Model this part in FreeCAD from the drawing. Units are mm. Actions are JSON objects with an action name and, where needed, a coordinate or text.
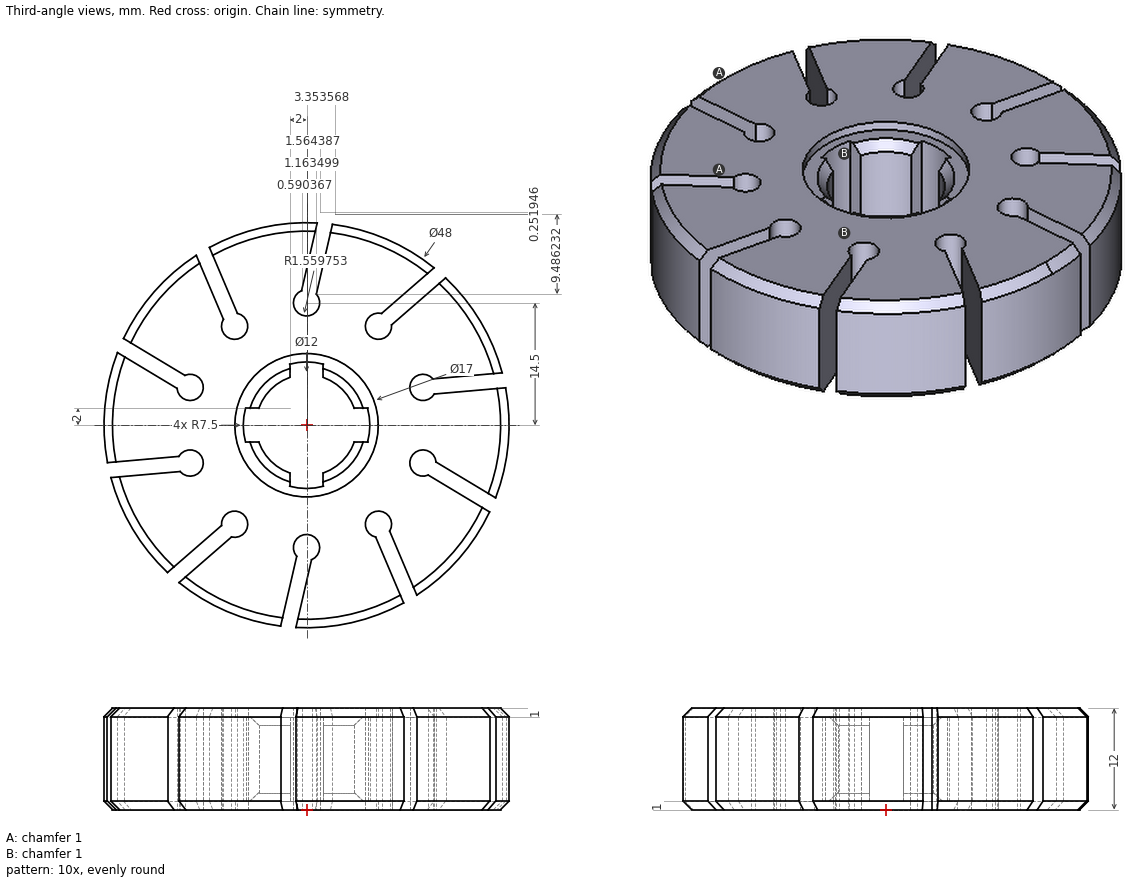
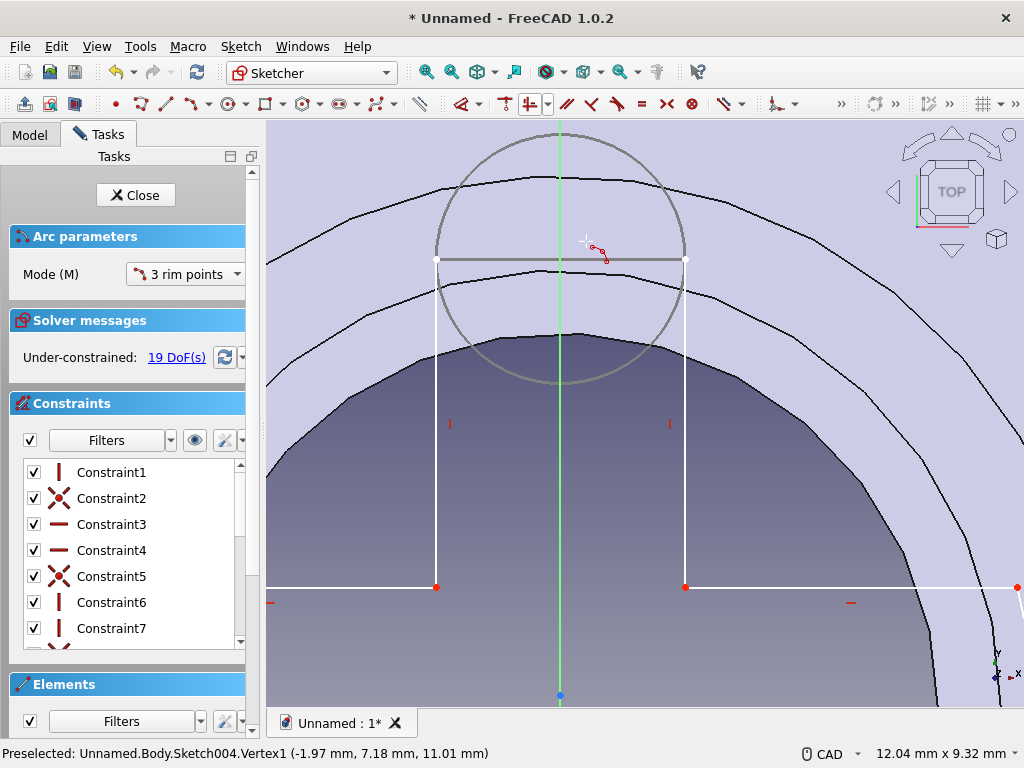
{"action": "left_click", "coordinate": [586, 240]}
{"action": "key", "text": "Escape"}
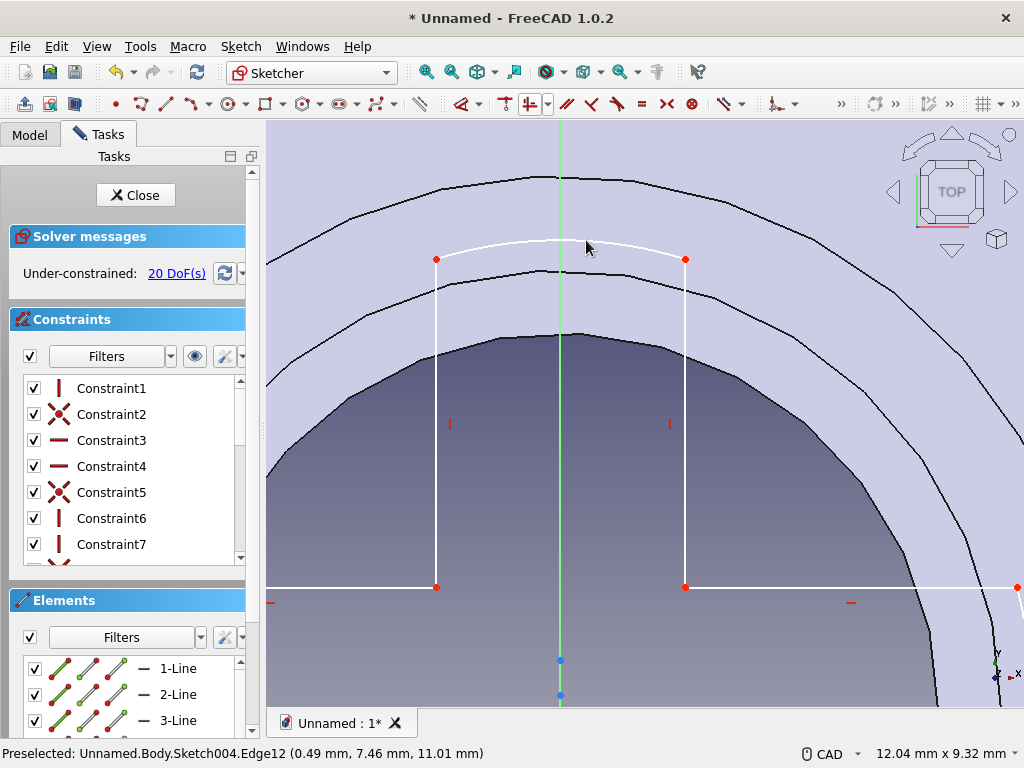
{"action": "scroll", "coordinate": [586, 240], "scroll_direction": "down", "scroll_amount": 5}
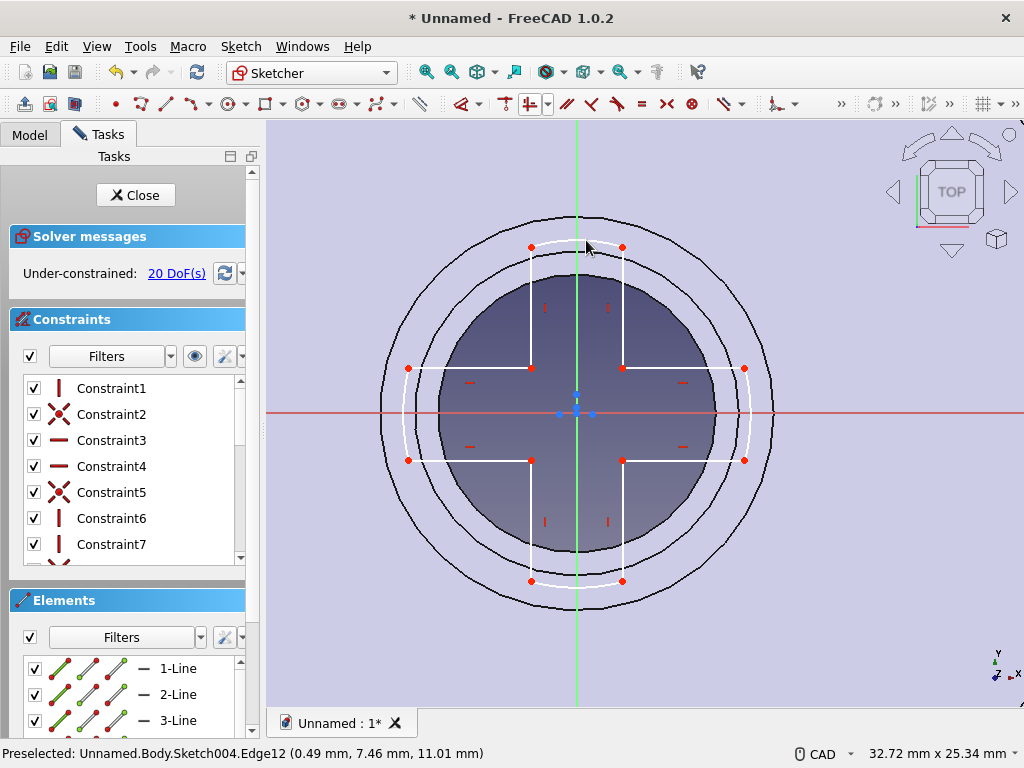
{"action": "left_click", "coordinate": [404, 396]}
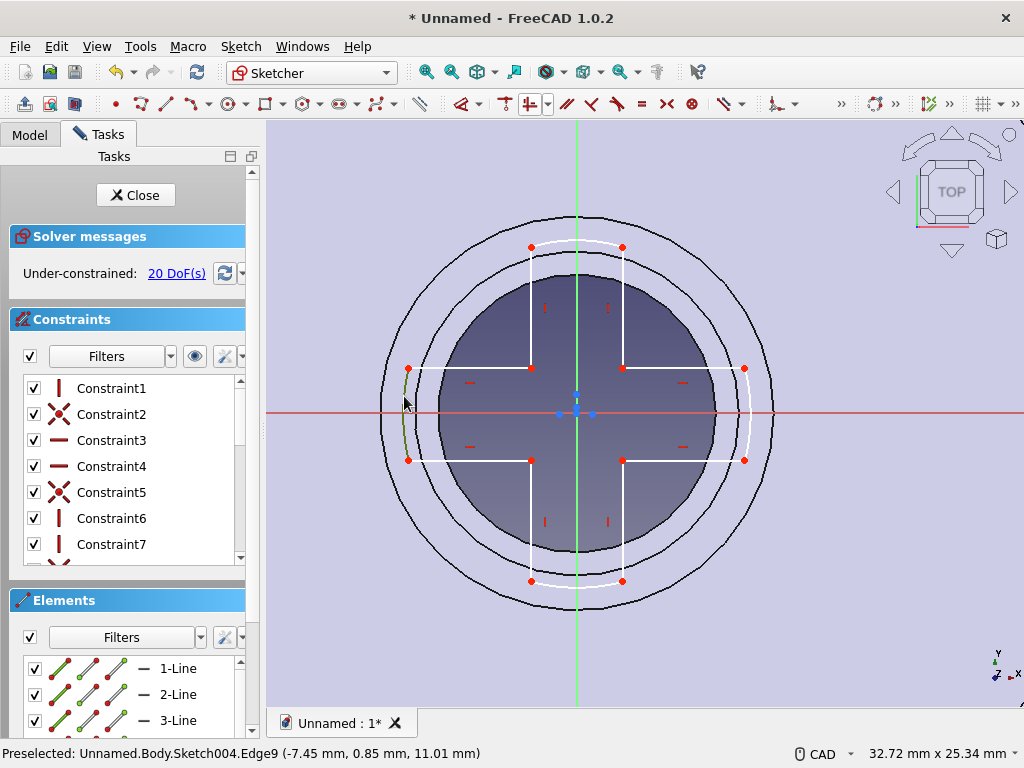
{"action": "left_click", "coordinate": [558, 587]}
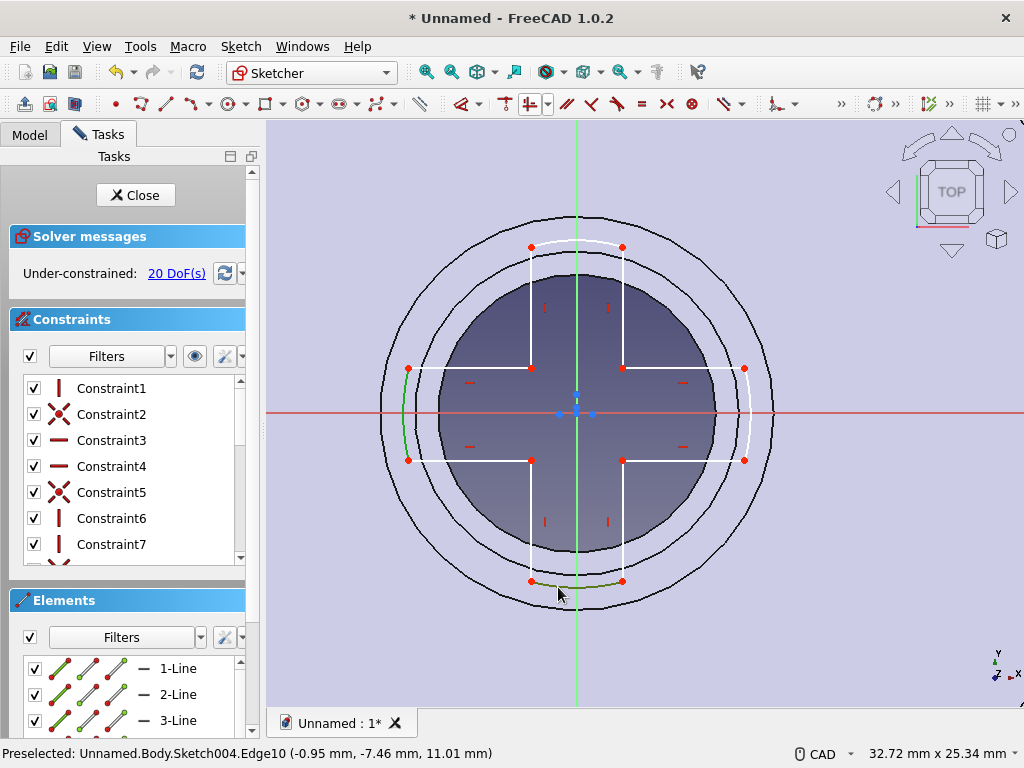
{"action": "left_click", "coordinate": [505, 104]}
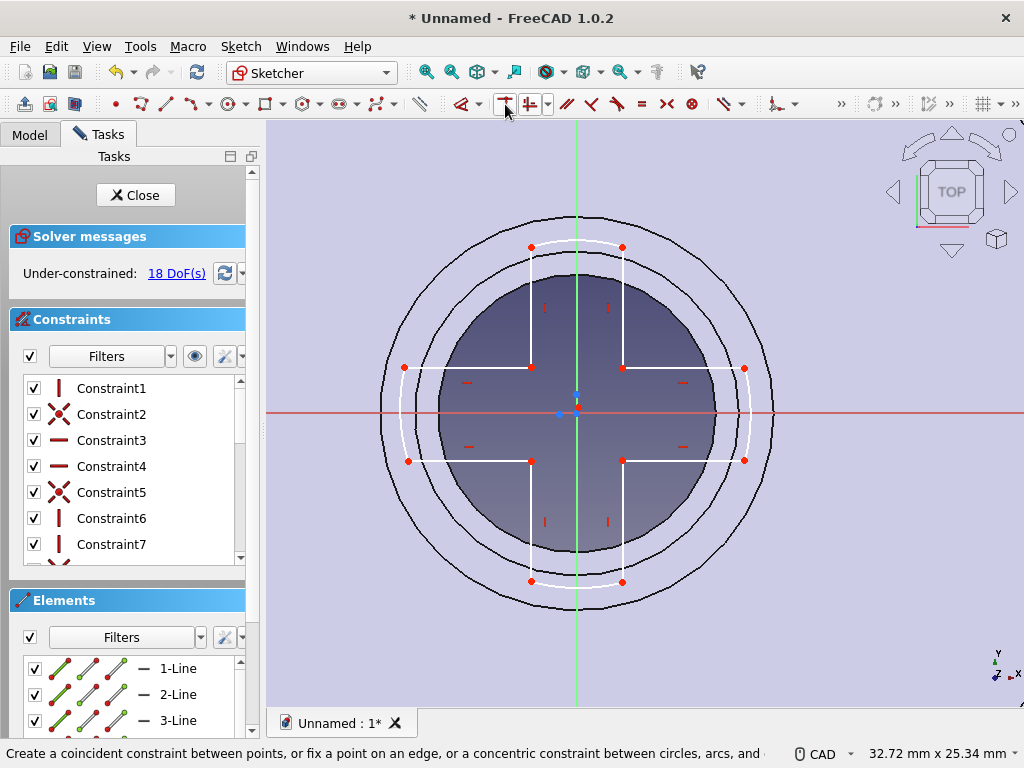
{"action": "left_click", "coordinate": [401, 396]}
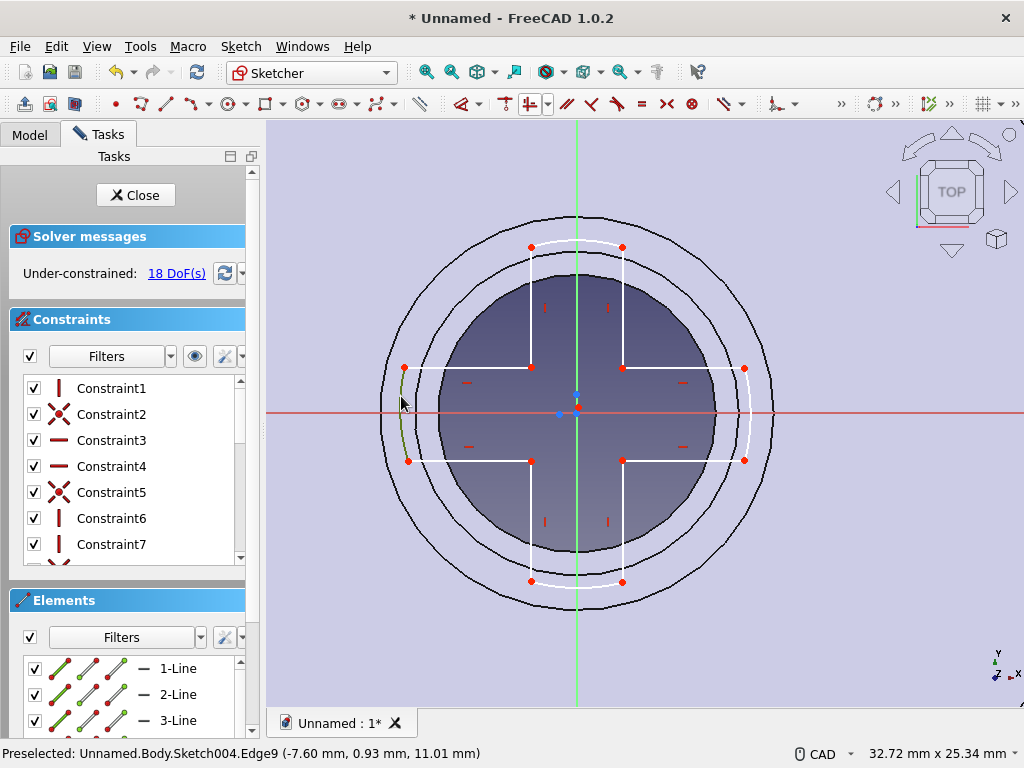
{"action": "left_click", "coordinate": [750, 433]}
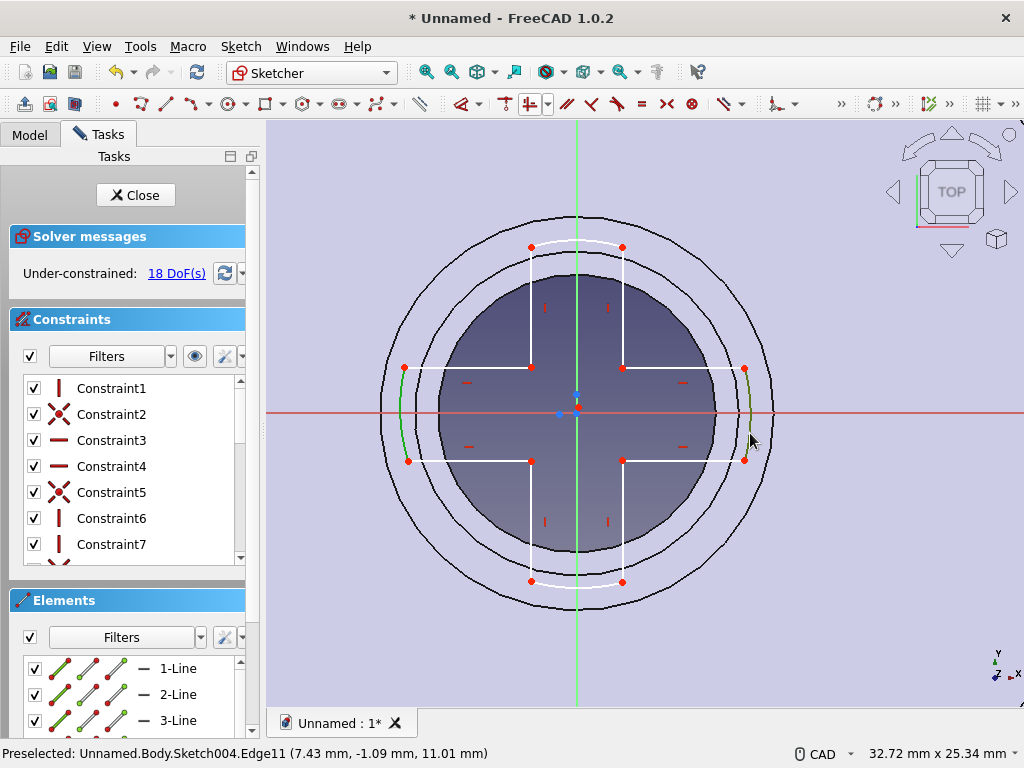
{"action": "left_click", "coordinate": [505, 104]}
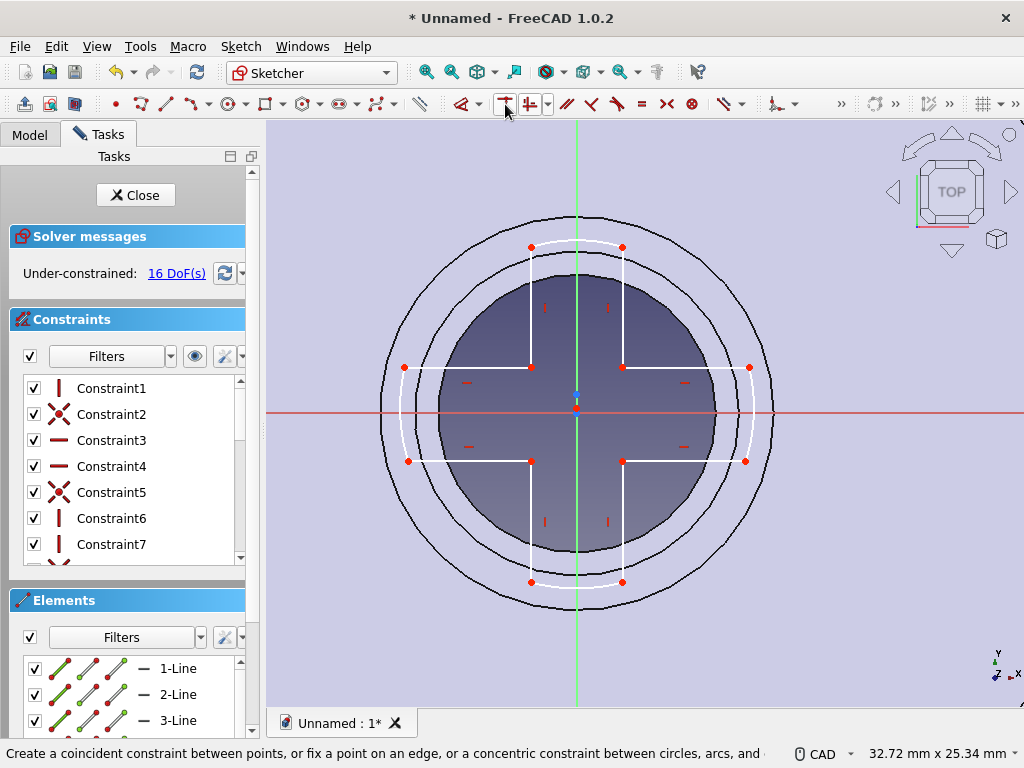
{"action": "left_click", "coordinate": [401, 396]}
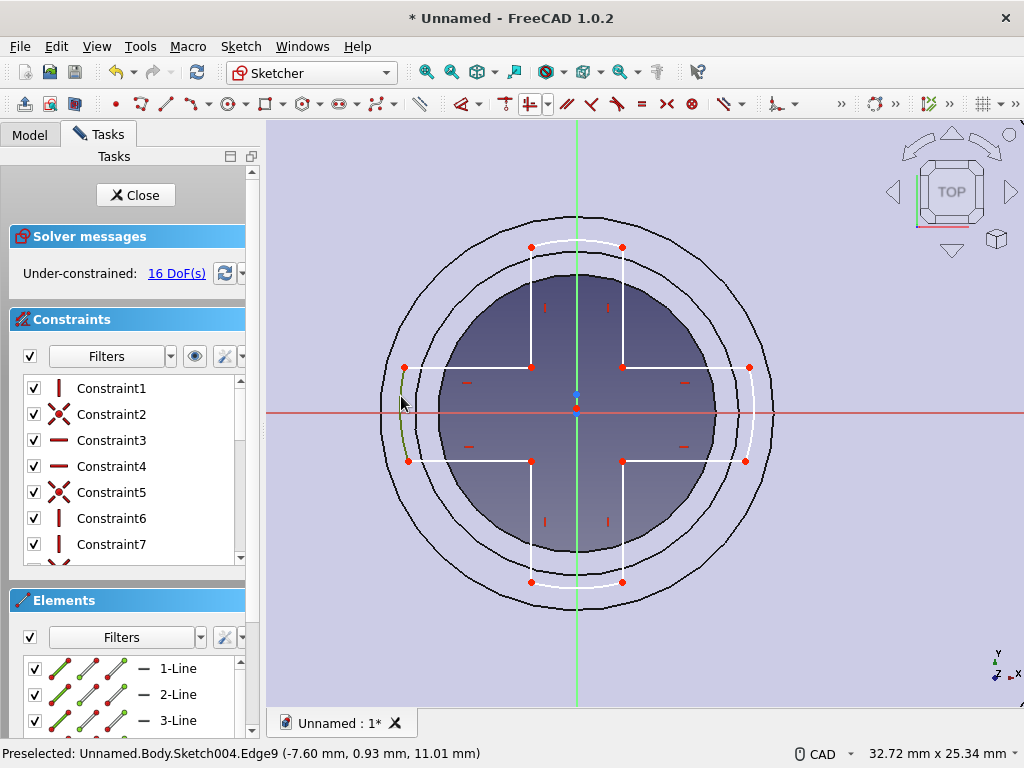
{"action": "left_click", "coordinate": [595, 241]}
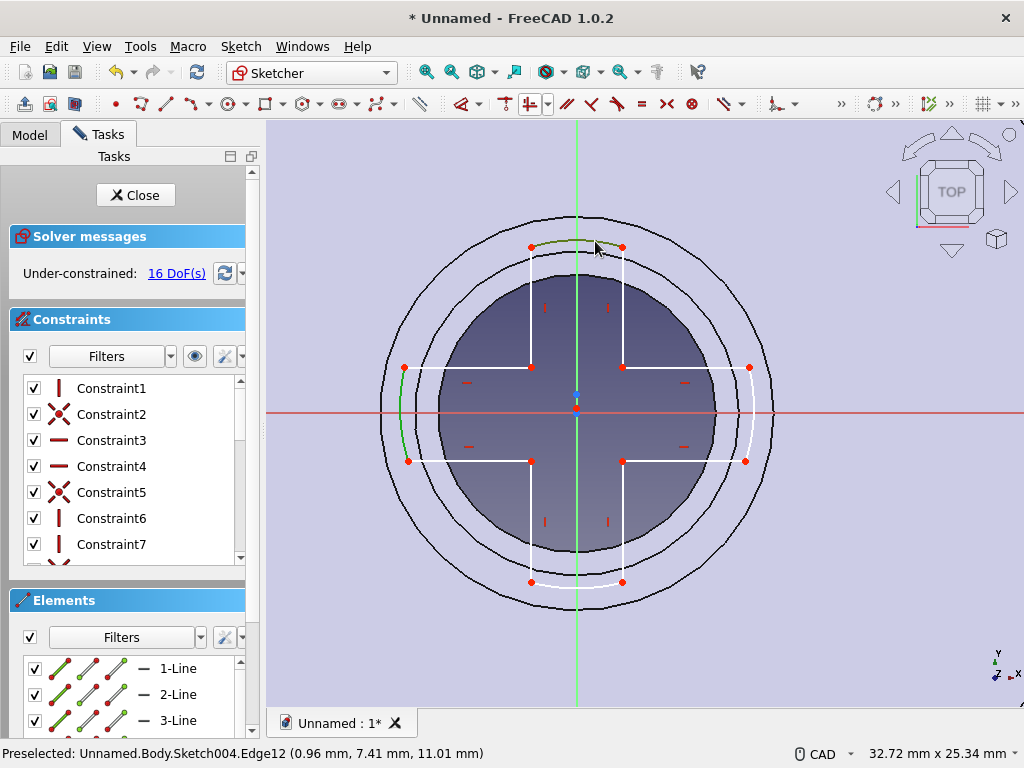
{"action": "left_click", "coordinate": [505, 104]}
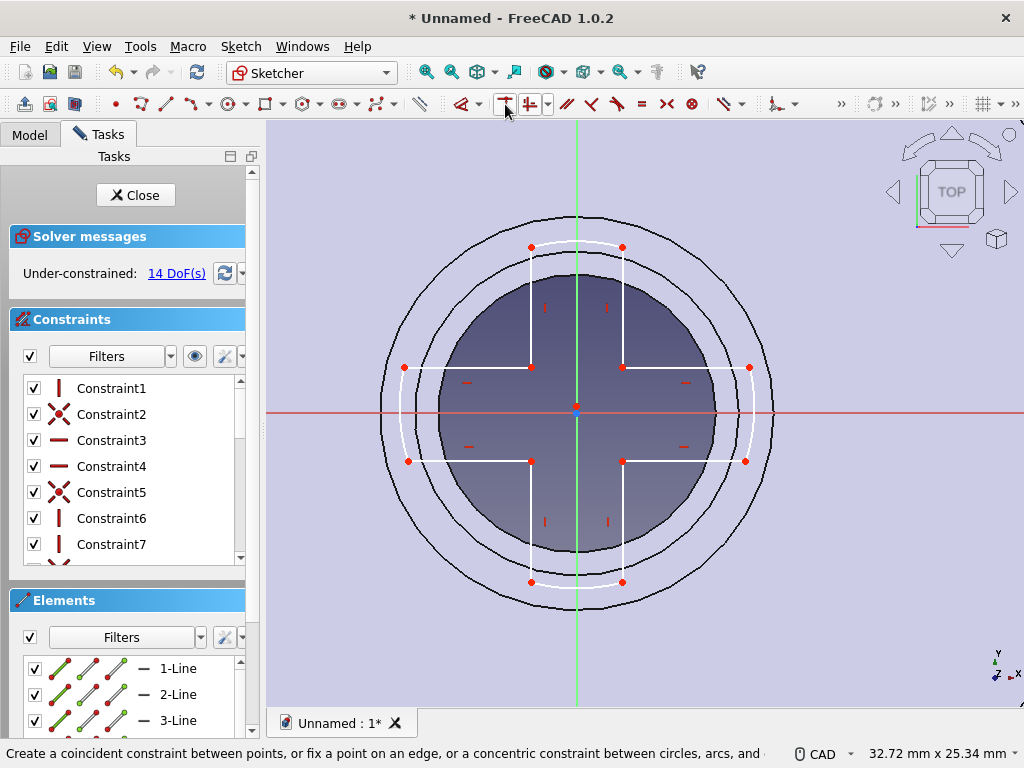
{"action": "left_click_drag", "start_coordinate": [567, 397], "coordinate": [587, 423]}